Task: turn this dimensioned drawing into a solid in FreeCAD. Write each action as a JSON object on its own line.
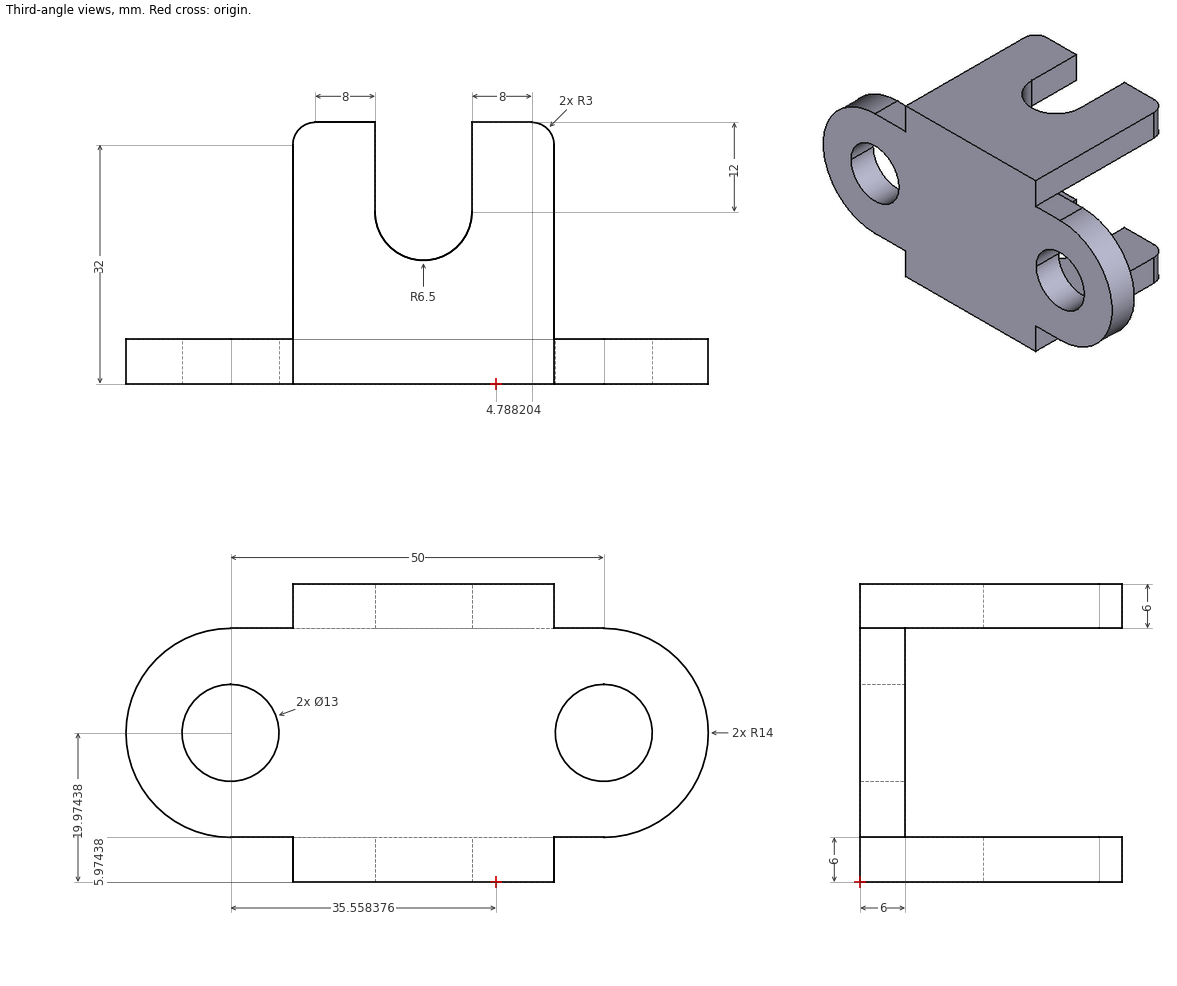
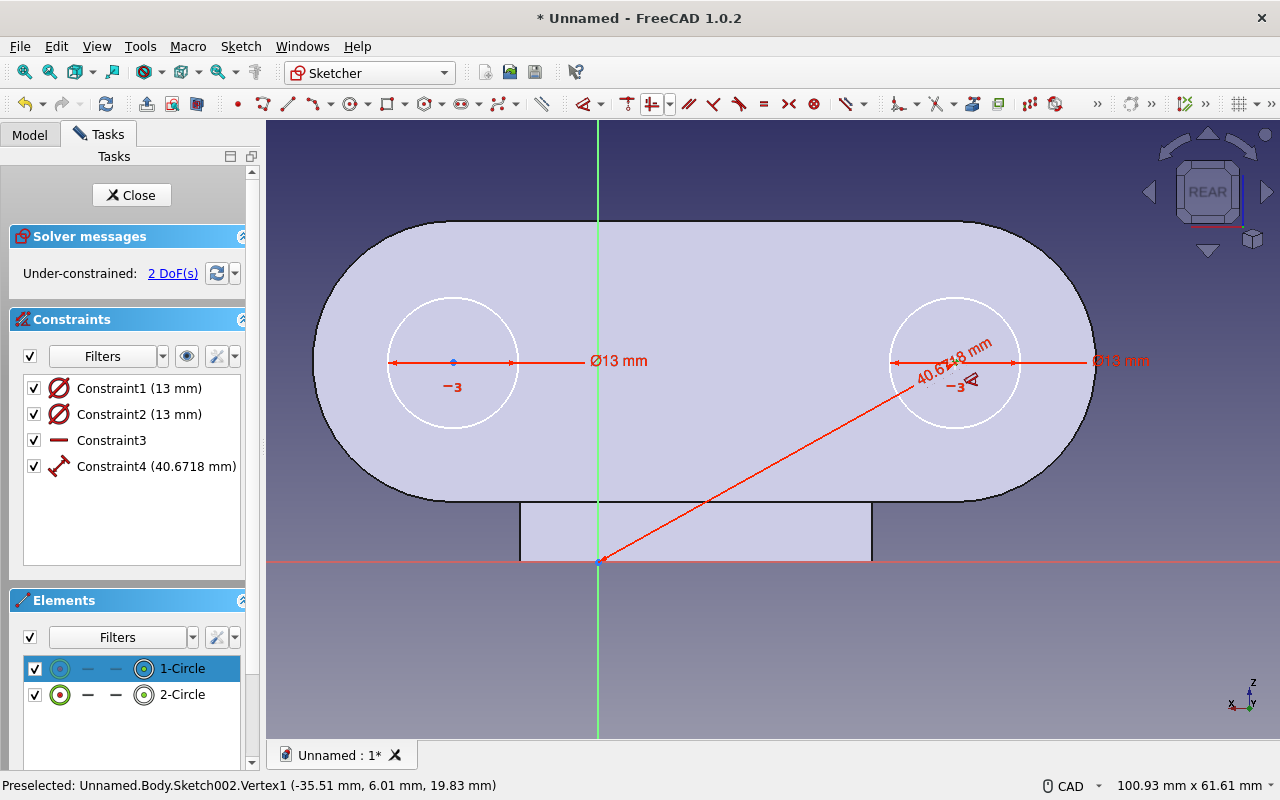
{"action": "left_click", "coordinate": [453, 363]}
{"action": "left_click", "coordinate": [704, 329]}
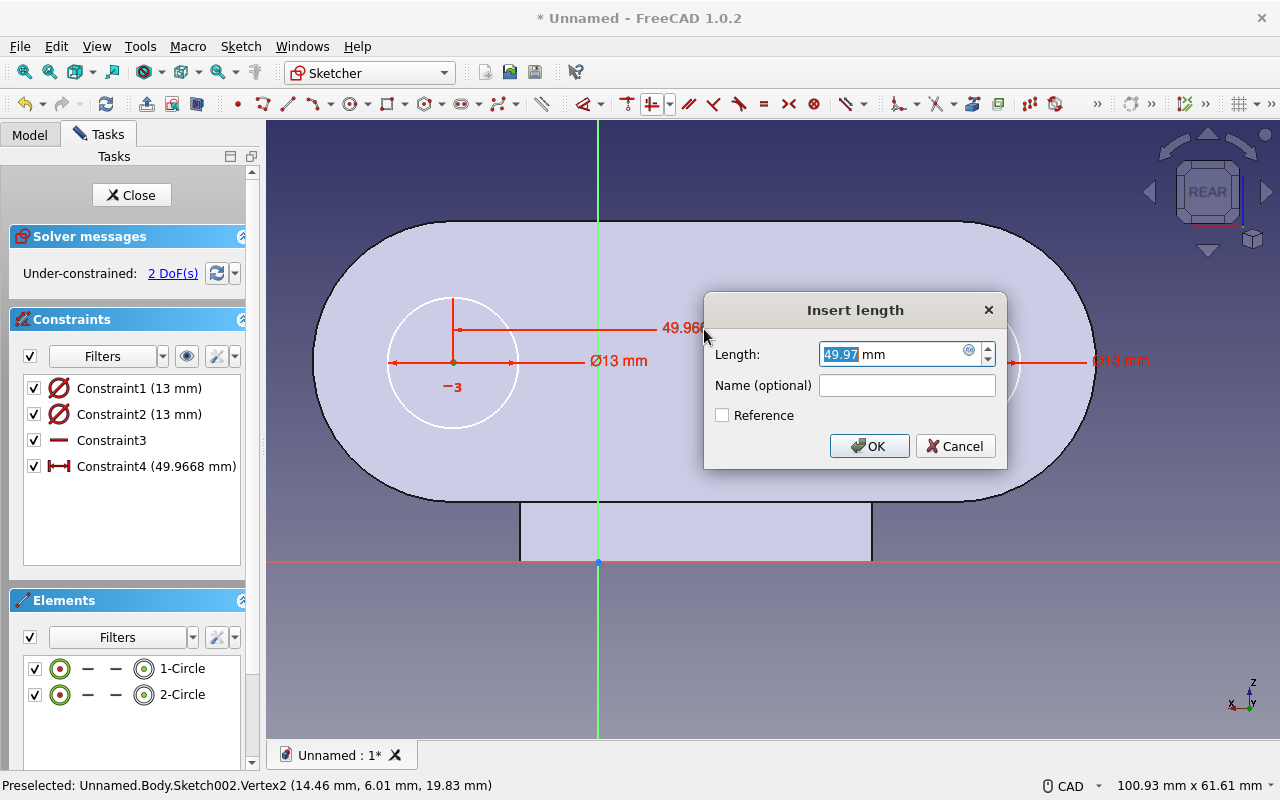
{"action": "type", "text": "50"}
{"action": "key", "text": "Return"}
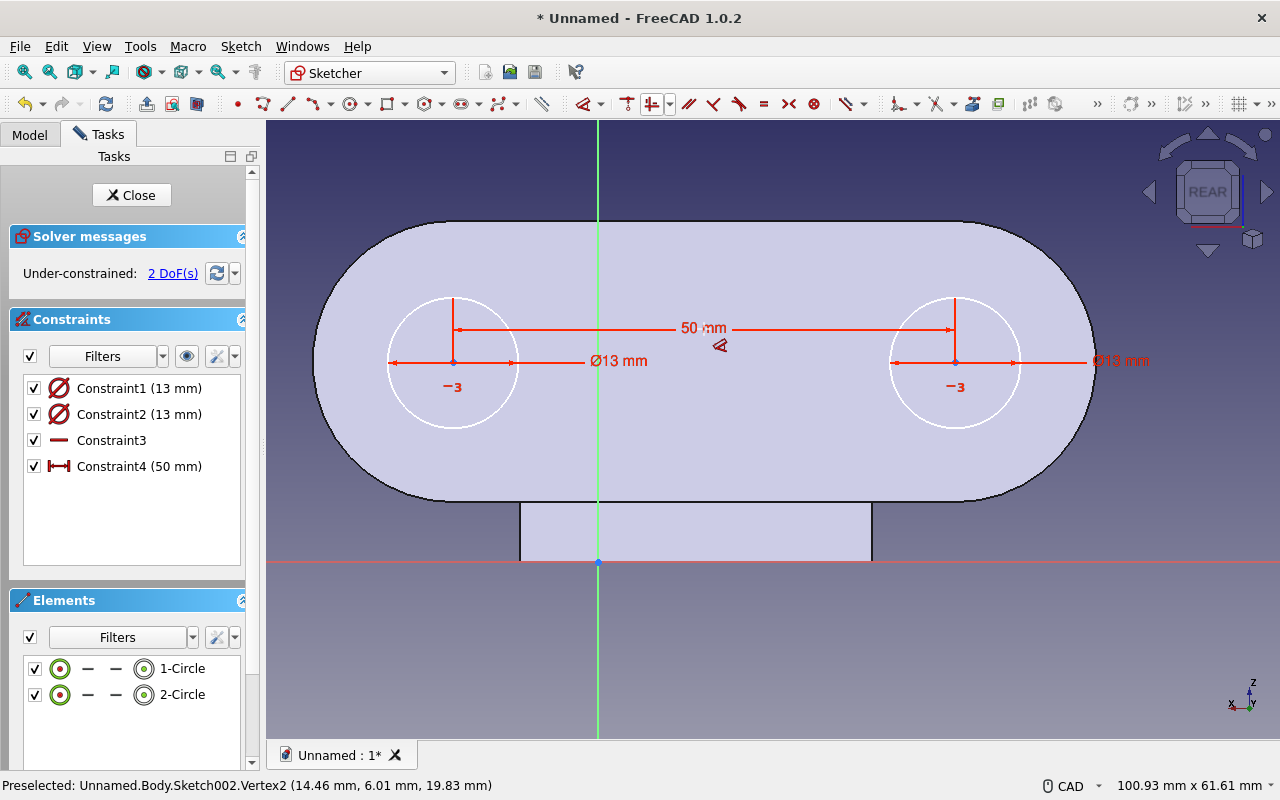
{"action": "left_click", "coordinate": [955, 363]}
{"action": "left_click", "coordinate": [989, 463]}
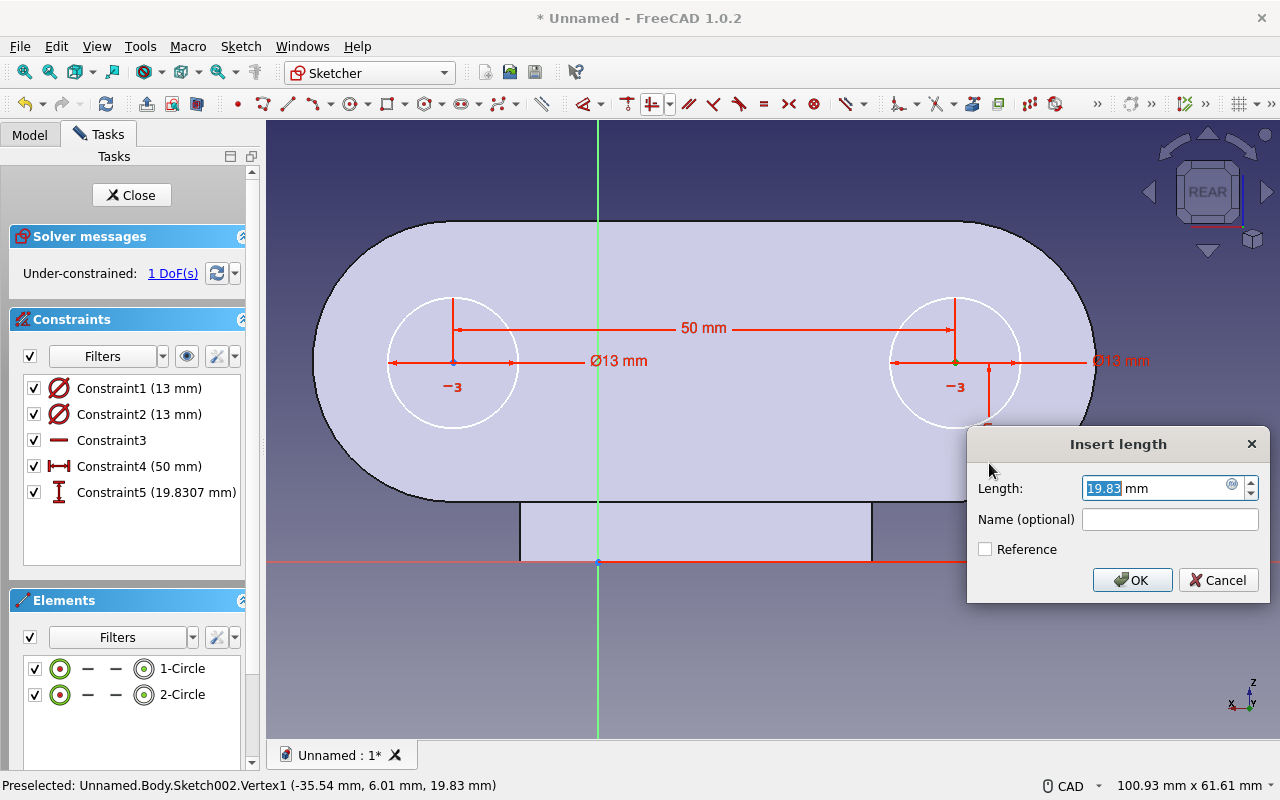
{"action": "type", "text": "19.97438"}
{"action": "key", "text": "Return"}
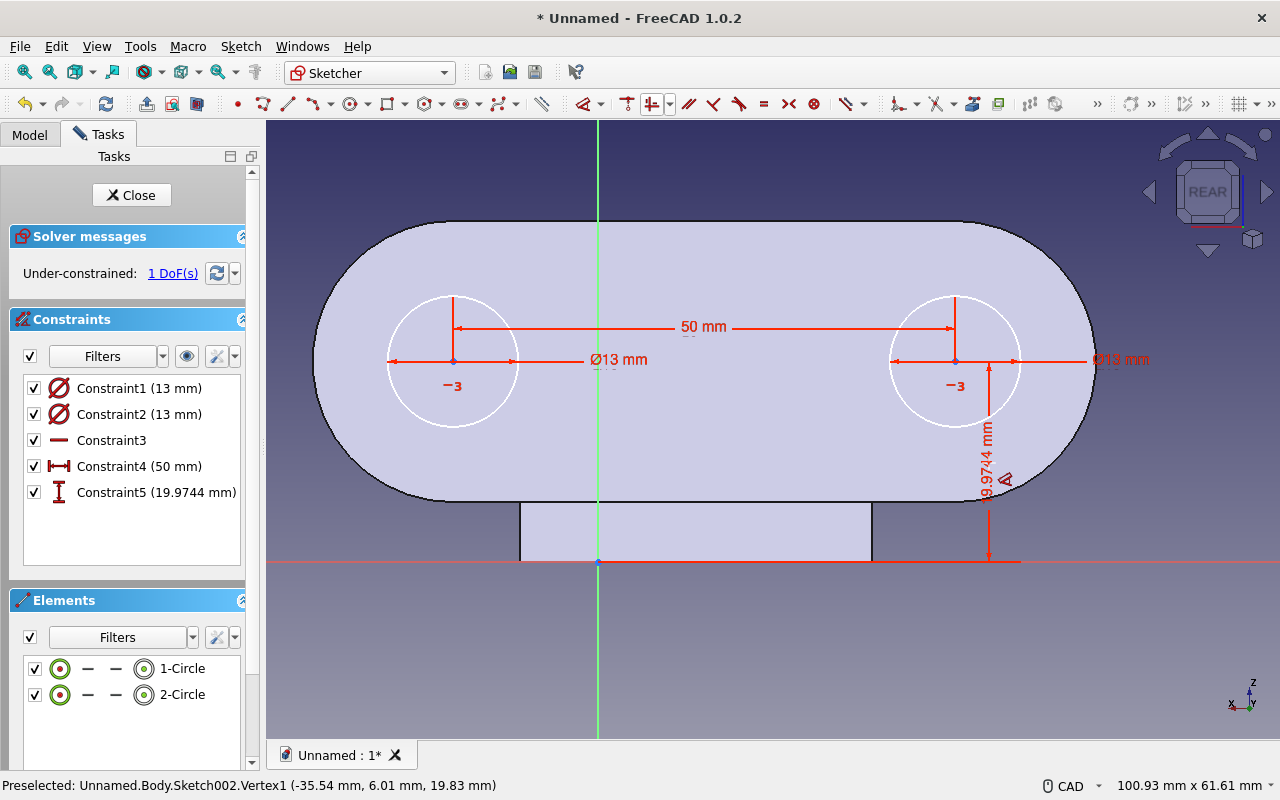
{"action": "left_click", "coordinate": [955, 362]}
{"action": "left_click", "coordinate": [777, 596]}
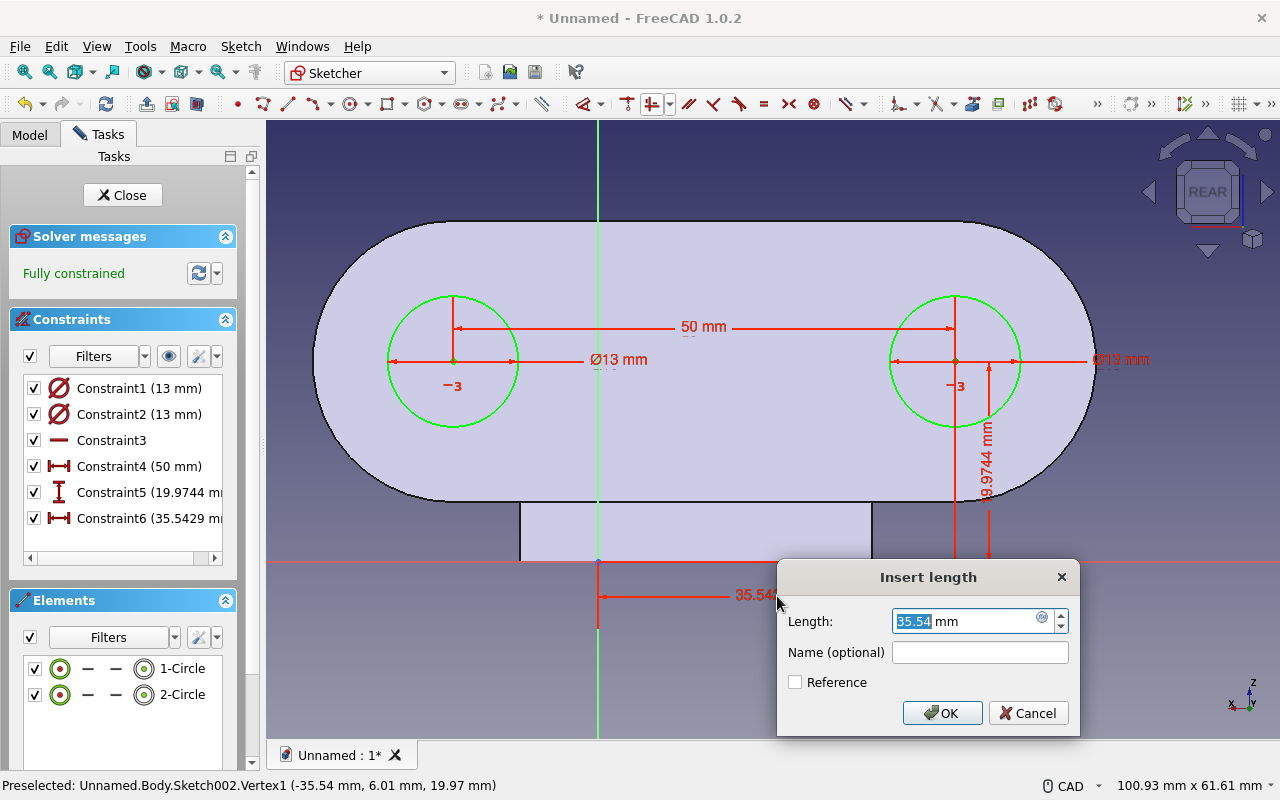
{"action": "type", "text": "35.558376"}
{"action": "key", "text": "Return"}
{"action": "key", "text": "Escape"}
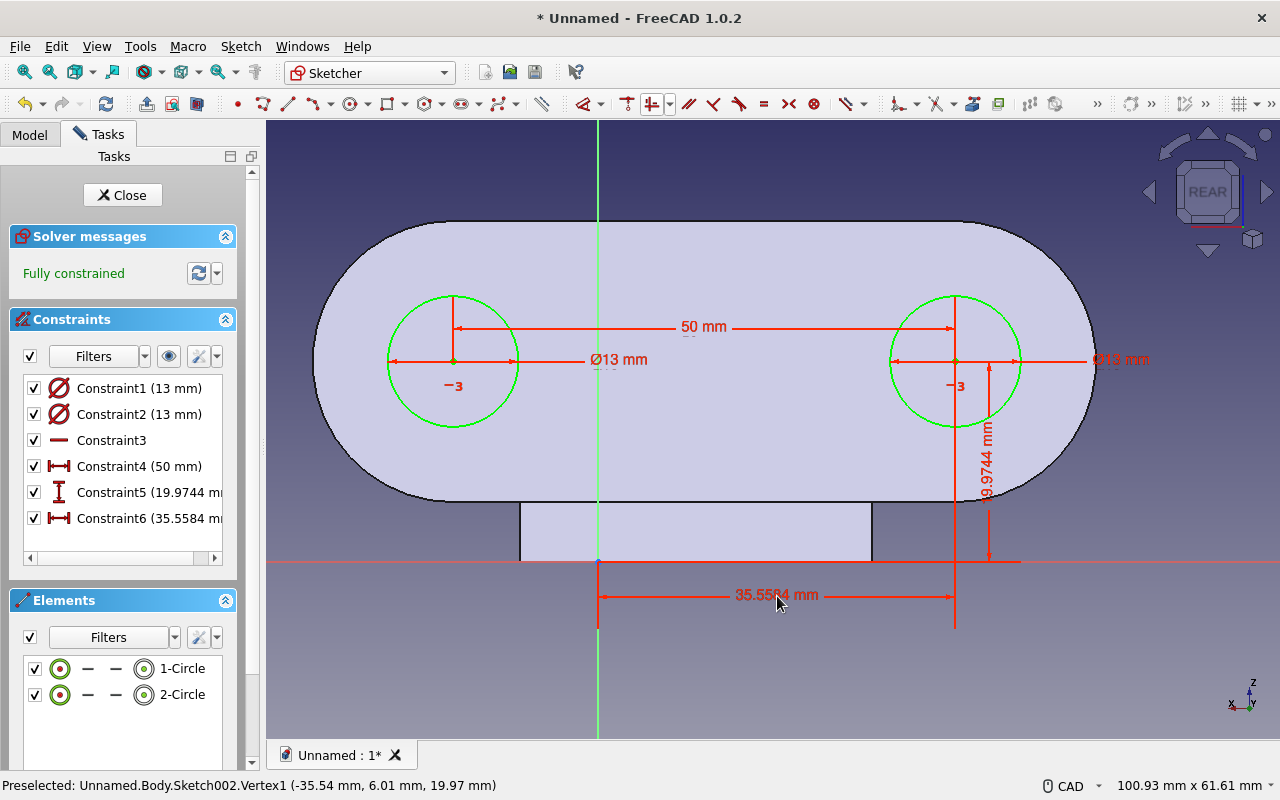
{"action": "left_click", "coordinate": [123, 195]}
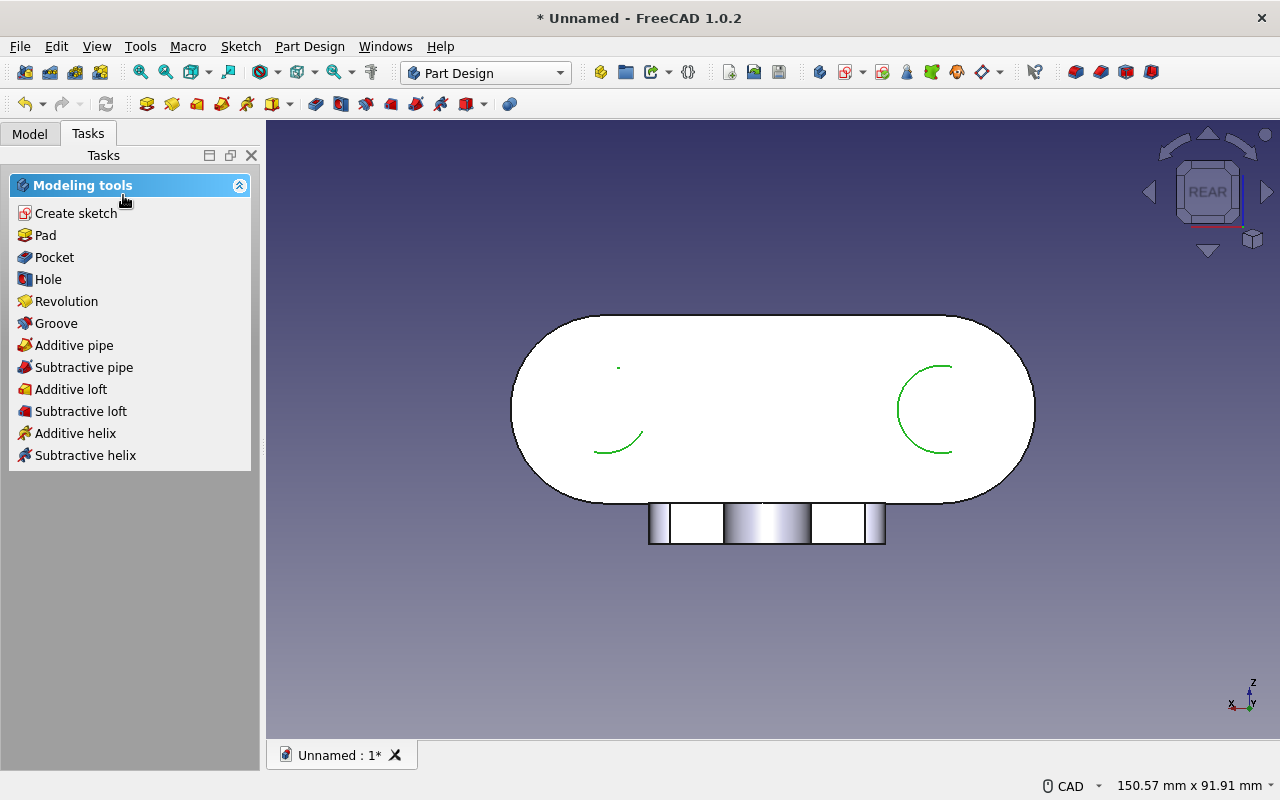
{"action": "left_click", "coordinate": [316, 104]}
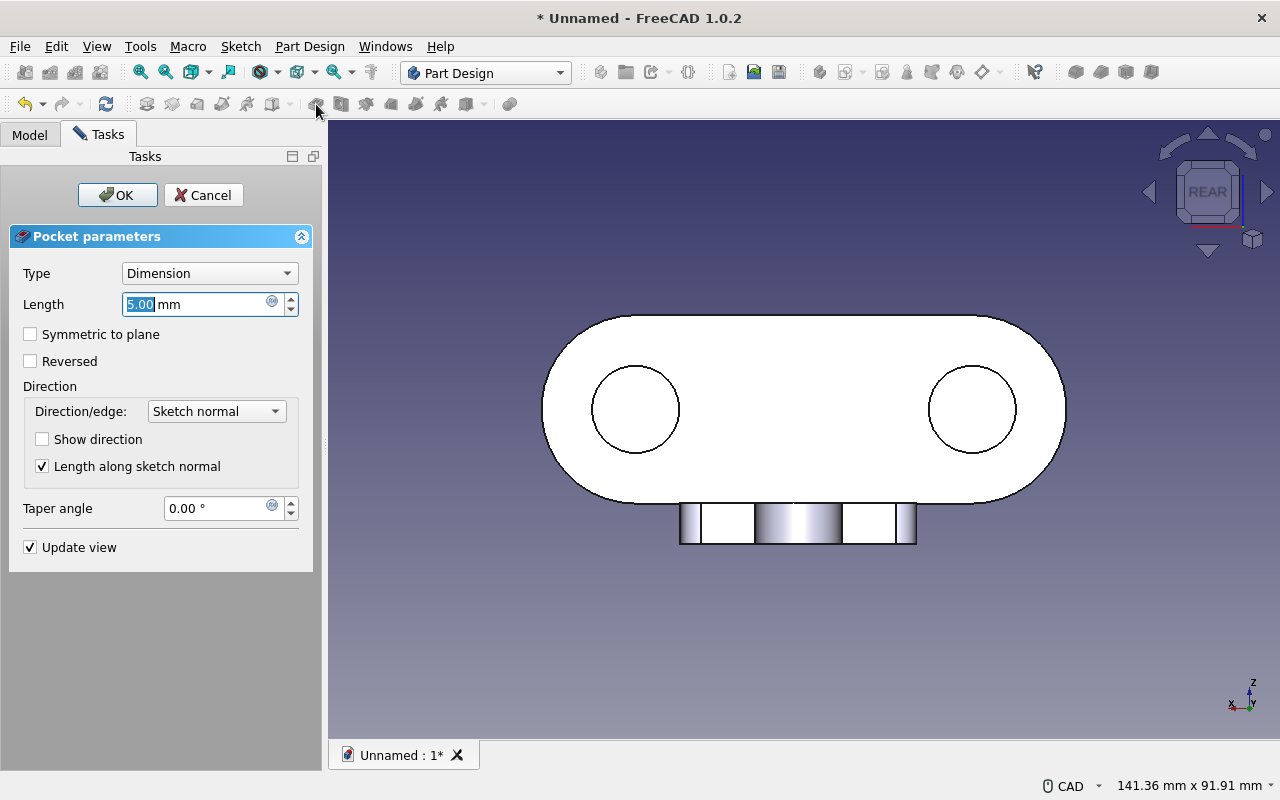
{"action": "left_click", "coordinate": [210, 274]}